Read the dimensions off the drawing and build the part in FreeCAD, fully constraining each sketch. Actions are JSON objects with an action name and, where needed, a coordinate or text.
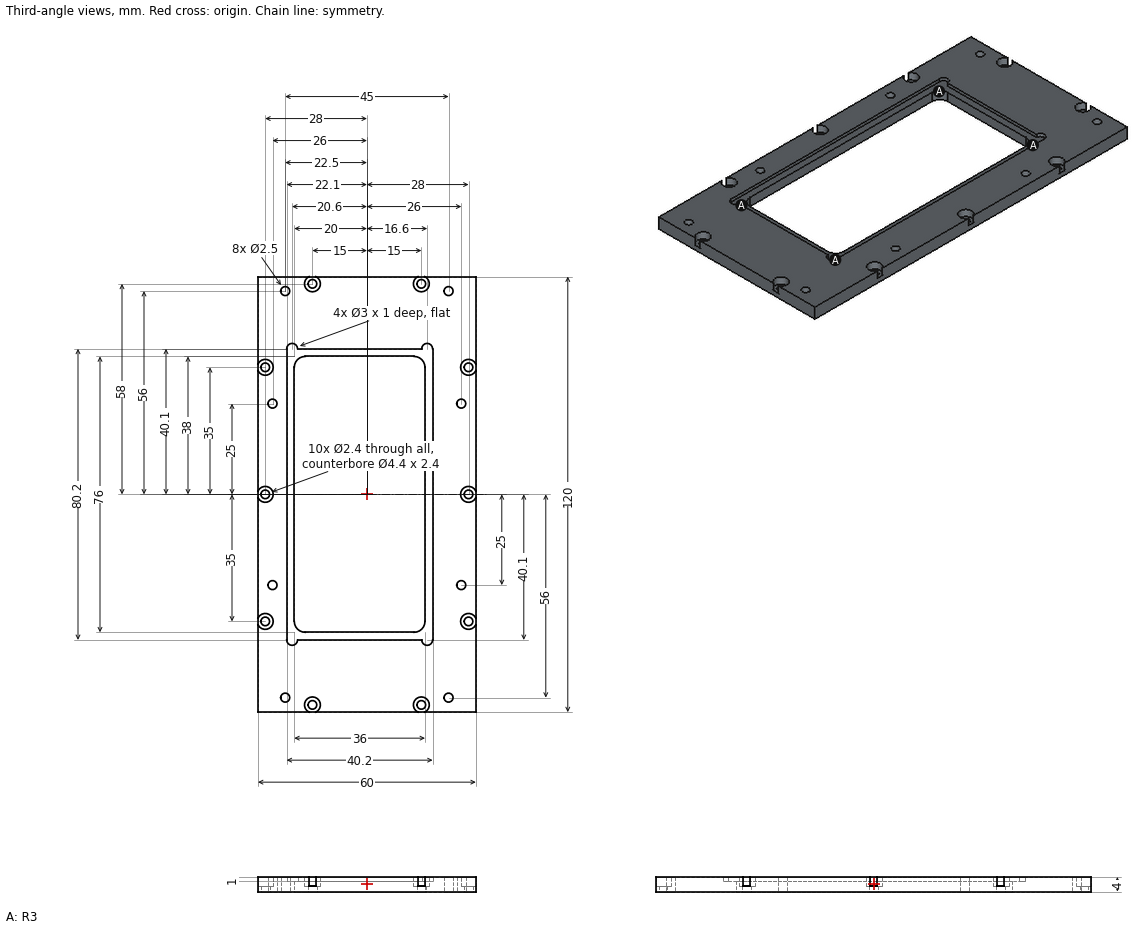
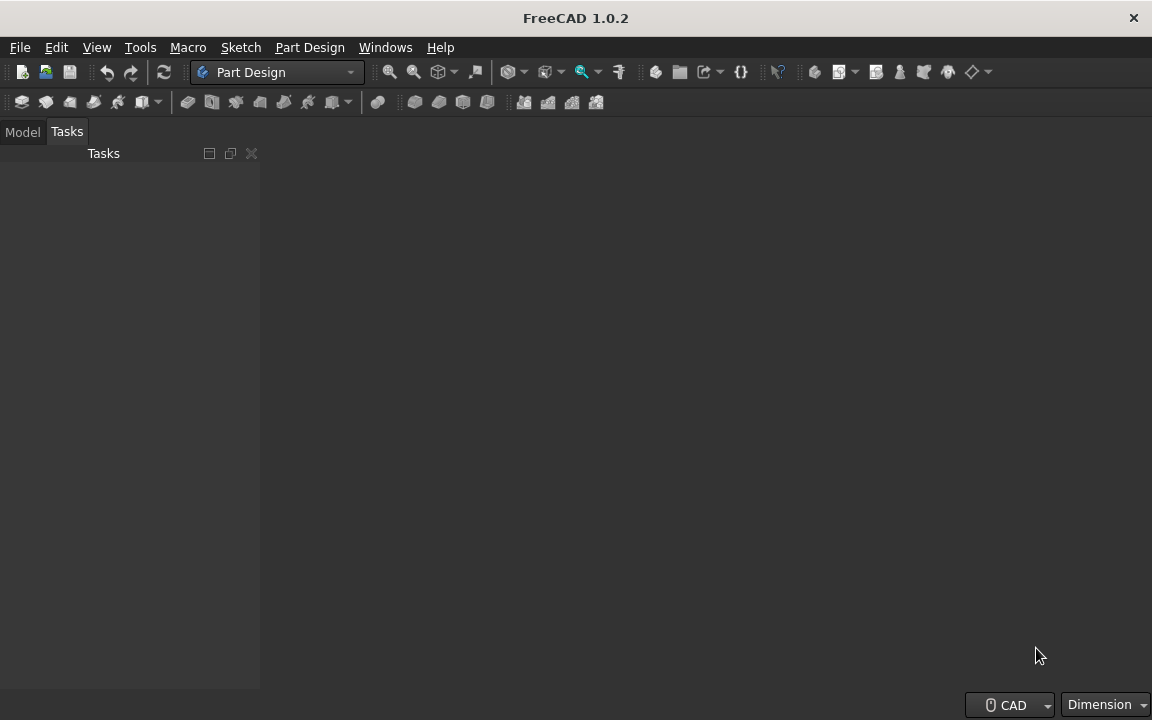
{"action": "key", "text": "ctrl+n"}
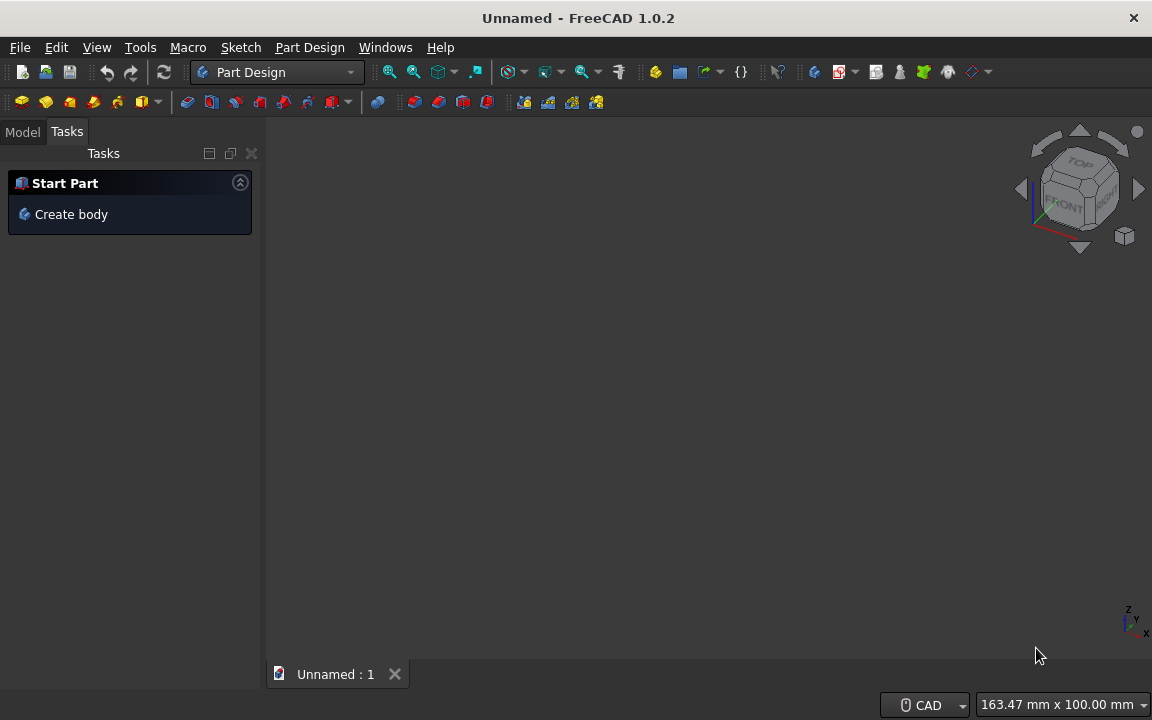
{"action": "left_click", "coordinate": [840, 72]}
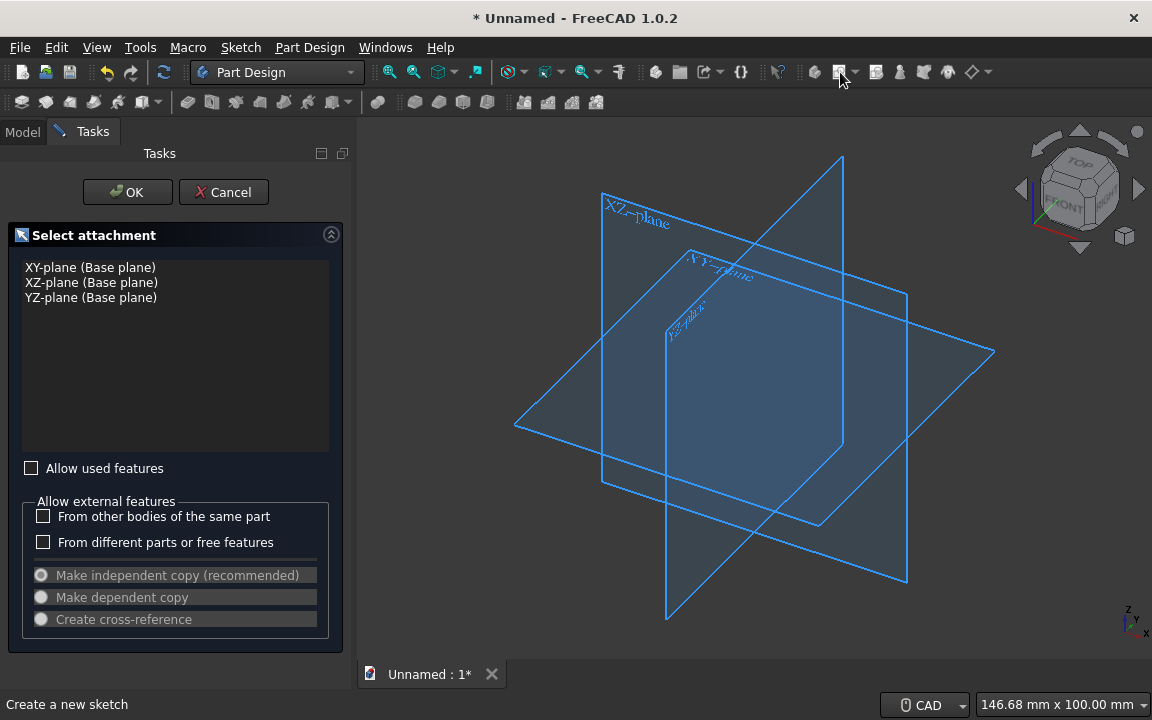
{"action": "left_click", "coordinate": [82, 268]}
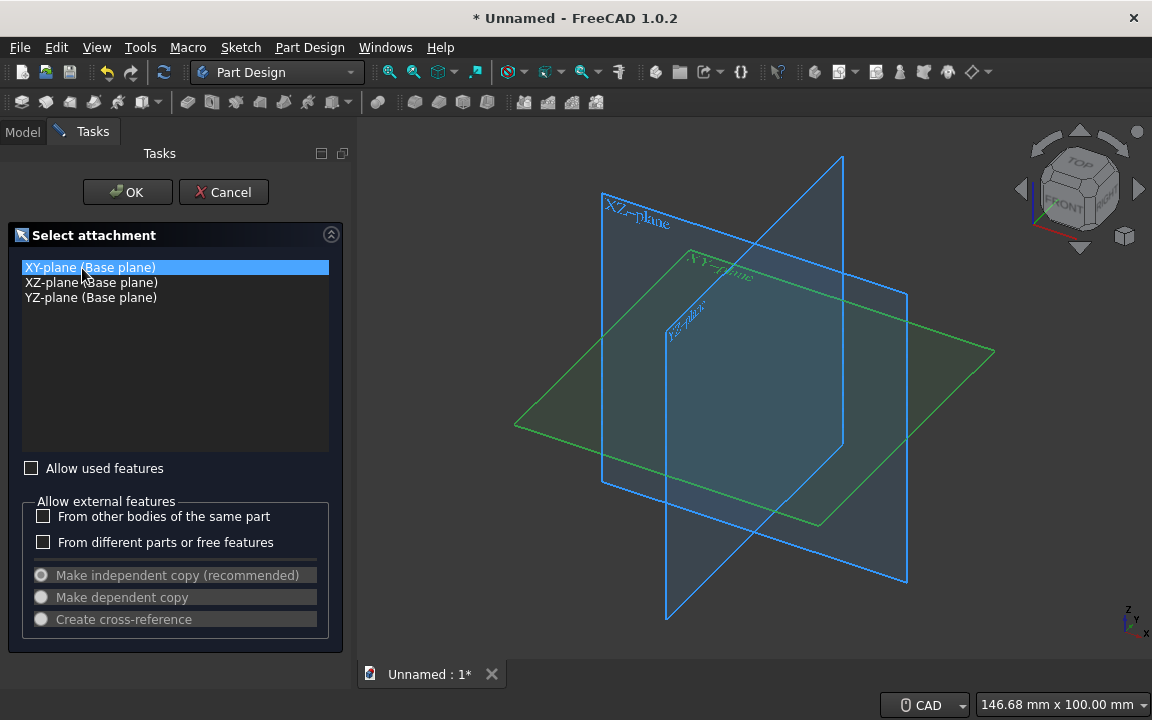
{"action": "left_click", "coordinate": [128, 192]}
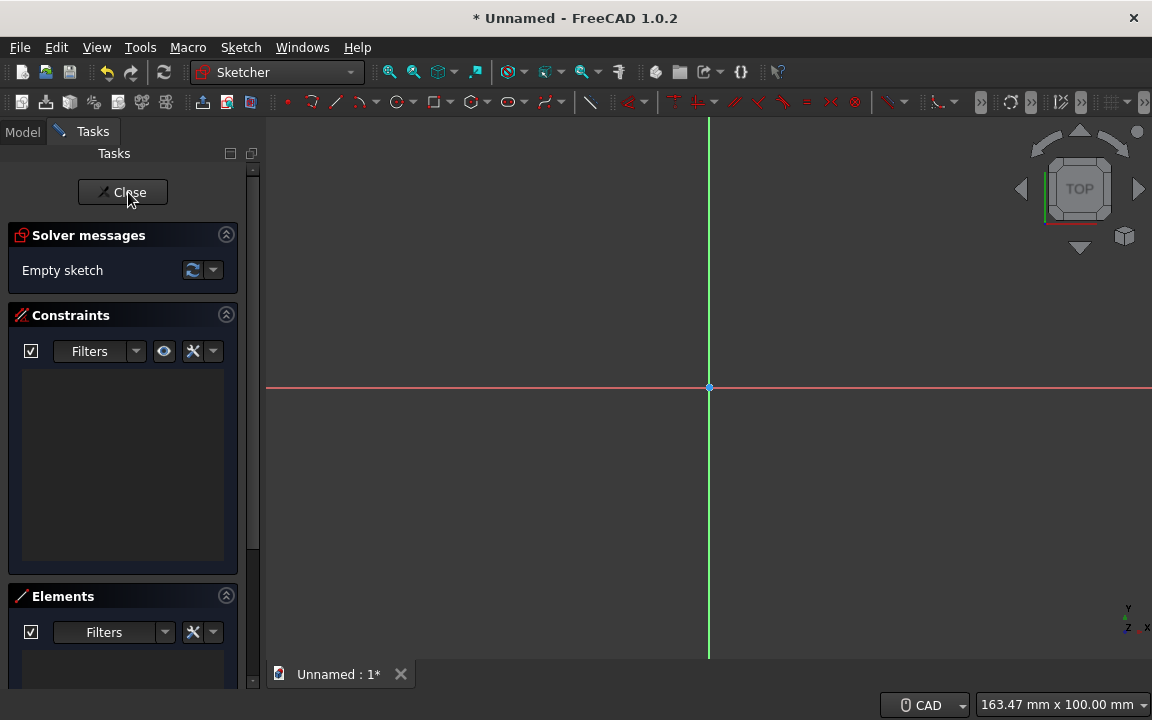
{"action": "scroll", "coordinate": [557, 388], "scroll_direction": "down", "scroll_amount": 3}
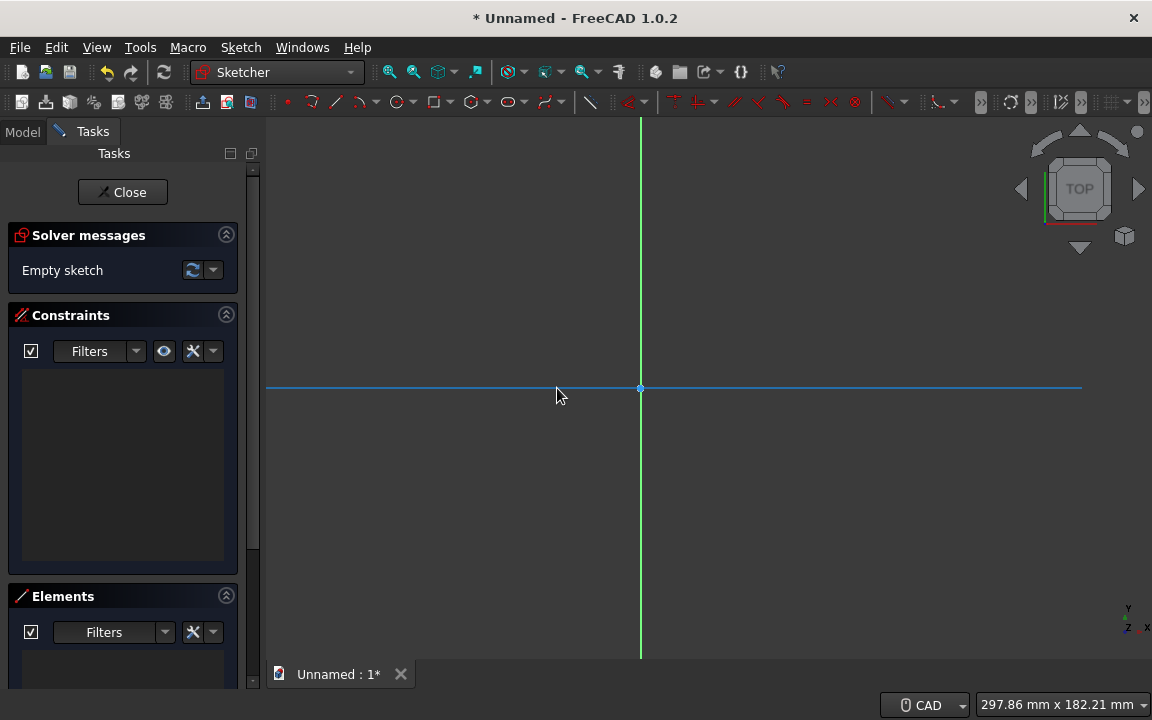
{"action": "key", "text": "g v"}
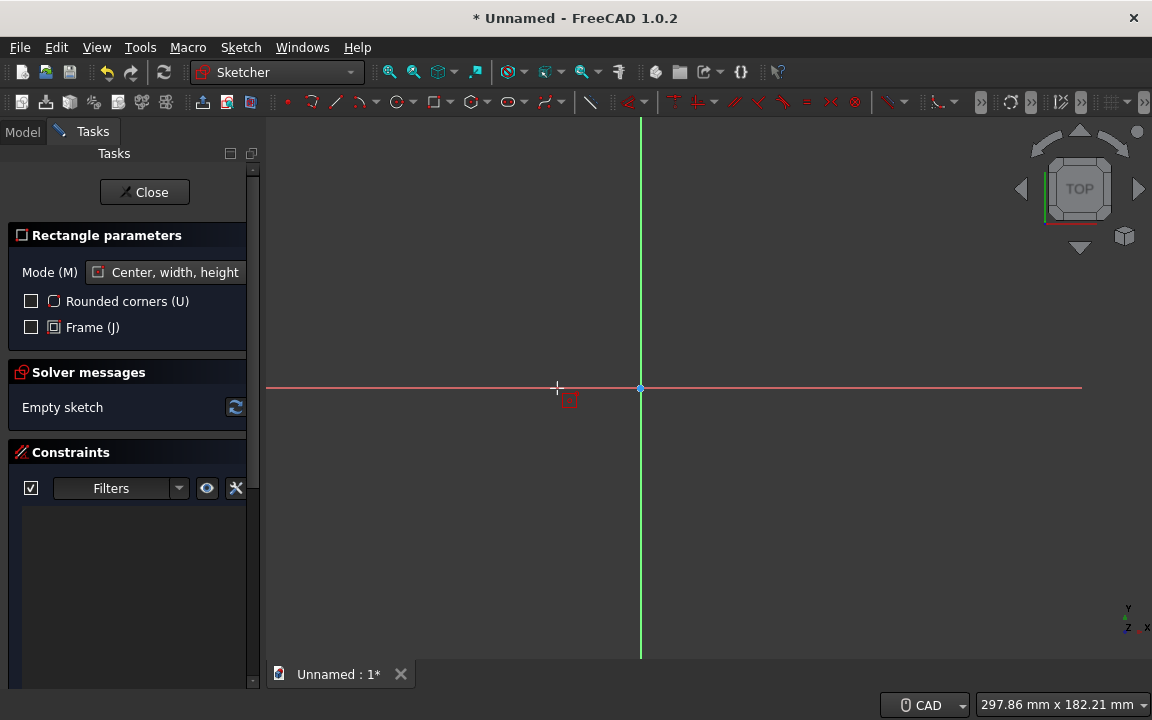
{"action": "left_click", "coordinate": [641, 388]}
{"action": "left_click", "coordinate": [730, 210]}
{"action": "key", "text": "Escape"}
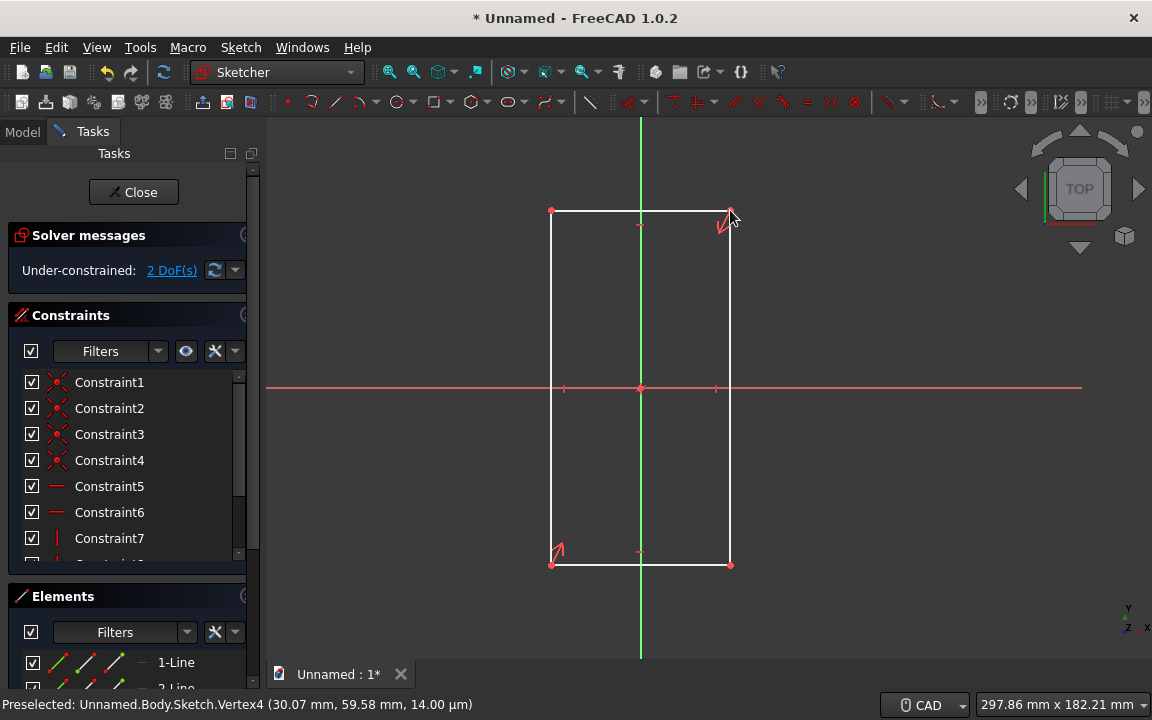
{"action": "key", "text": "d"}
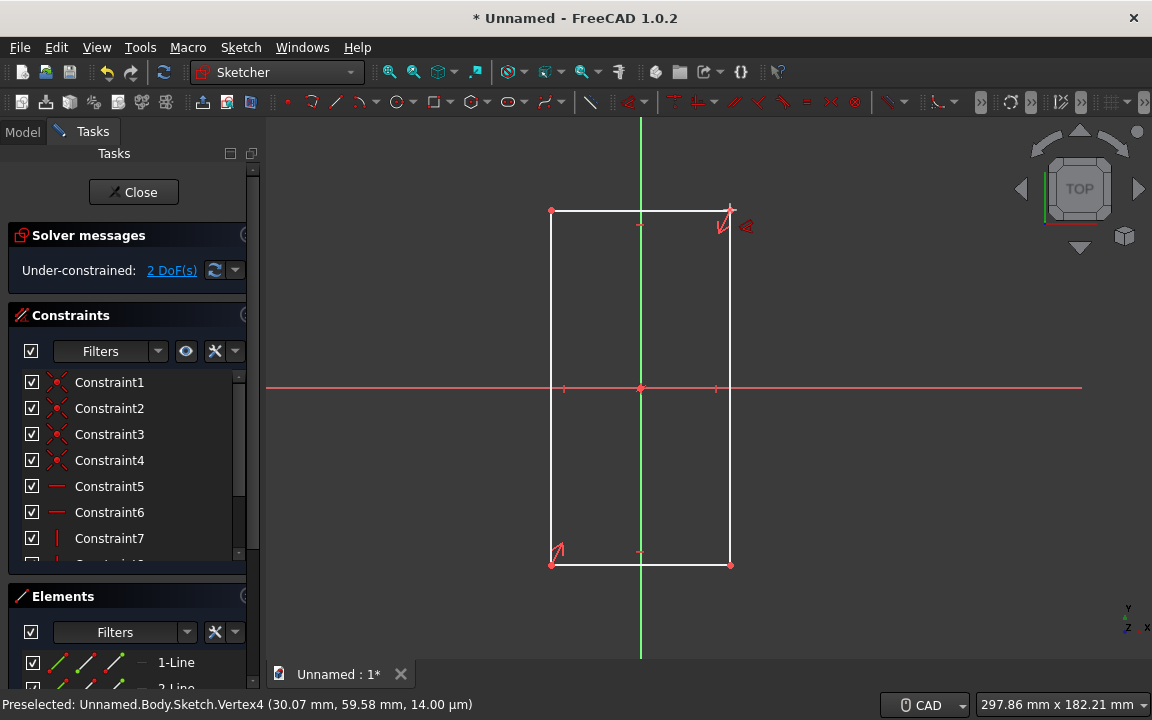
{"action": "left_click", "coordinate": [605, 565]}
{"action": "left_click", "coordinate": [599, 599]}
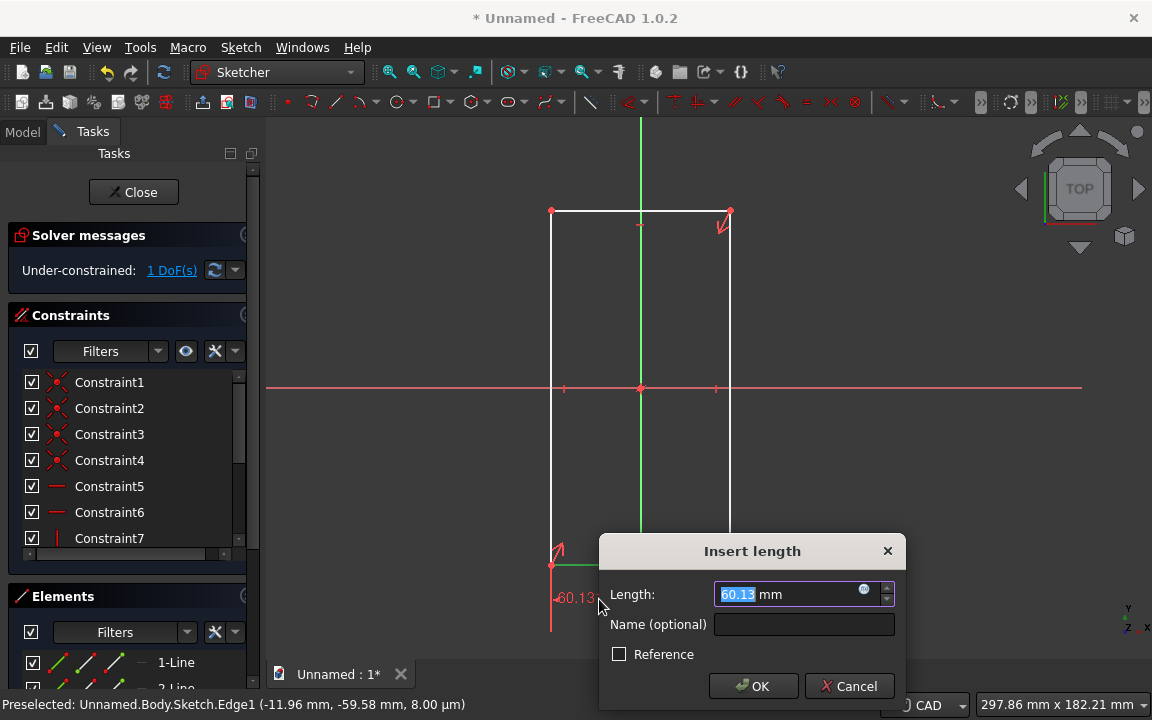
{"action": "type", "text": "60"}
{"action": "key", "text": "Return"}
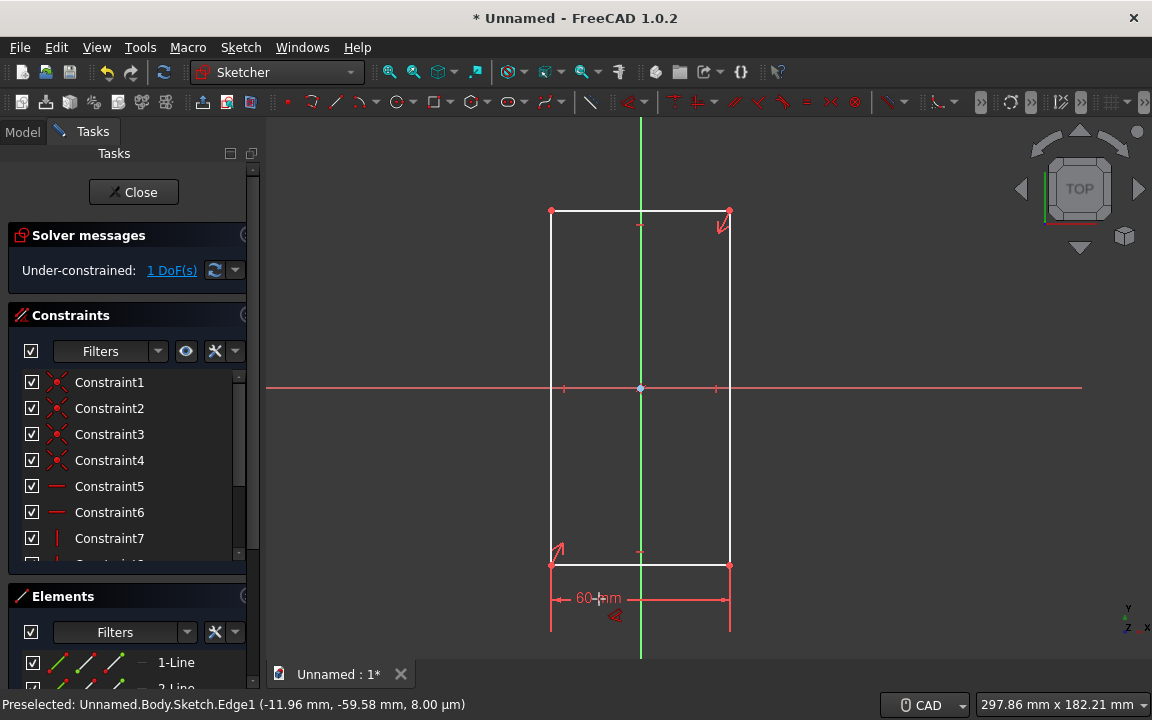
{"action": "left_click", "coordinate": [730, 459]}
{"action": "left_click", "coordinate": [764, 307]}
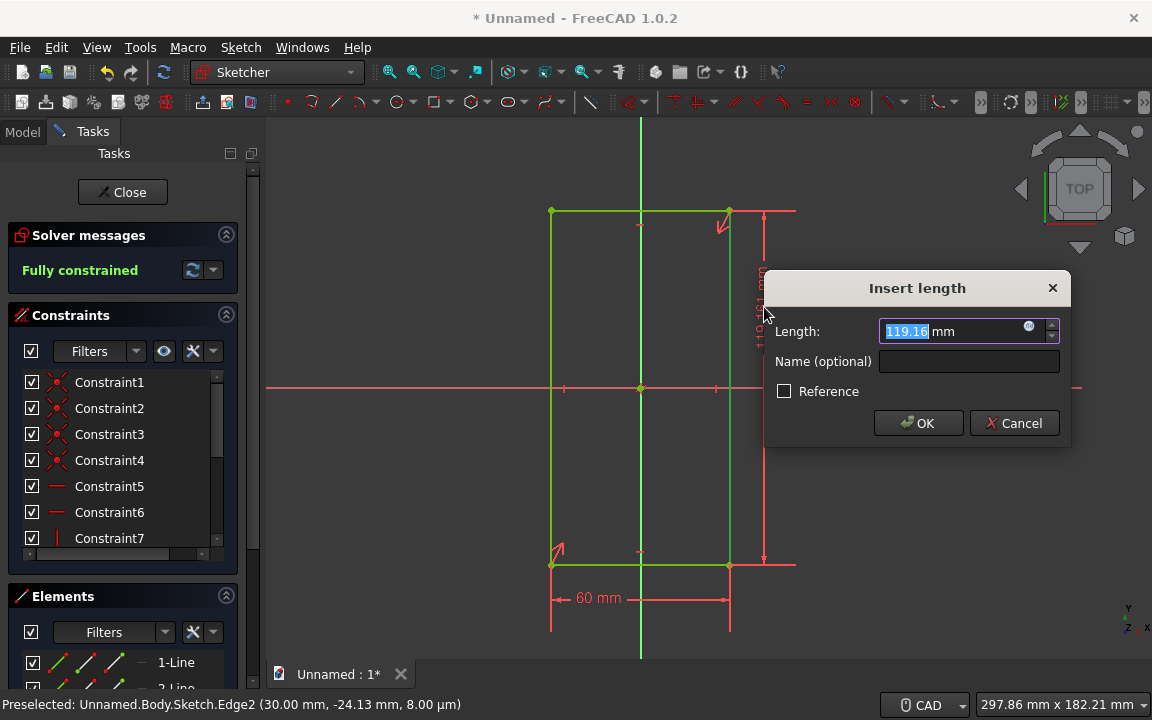
{"action": "type", "text": "120"}
{"action": "key", "text": "Return"}
{"action": "key", "text": "Escape"}